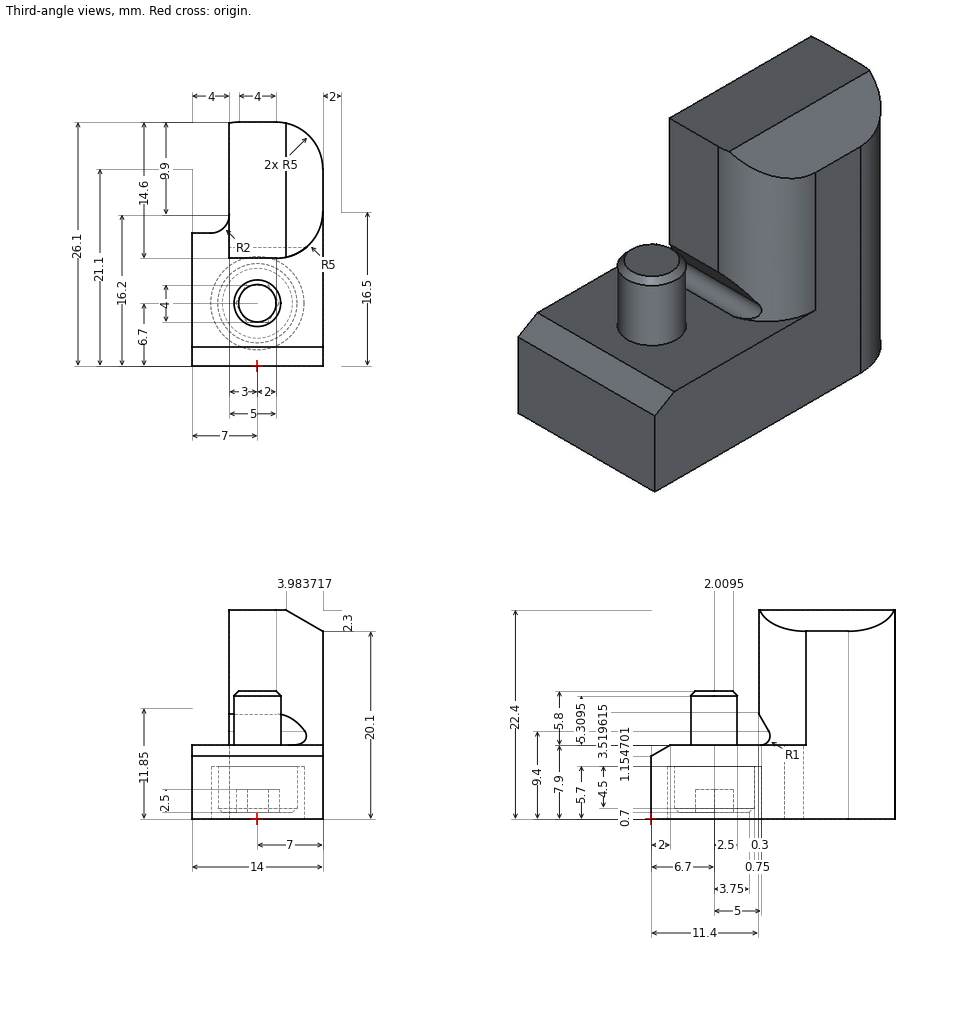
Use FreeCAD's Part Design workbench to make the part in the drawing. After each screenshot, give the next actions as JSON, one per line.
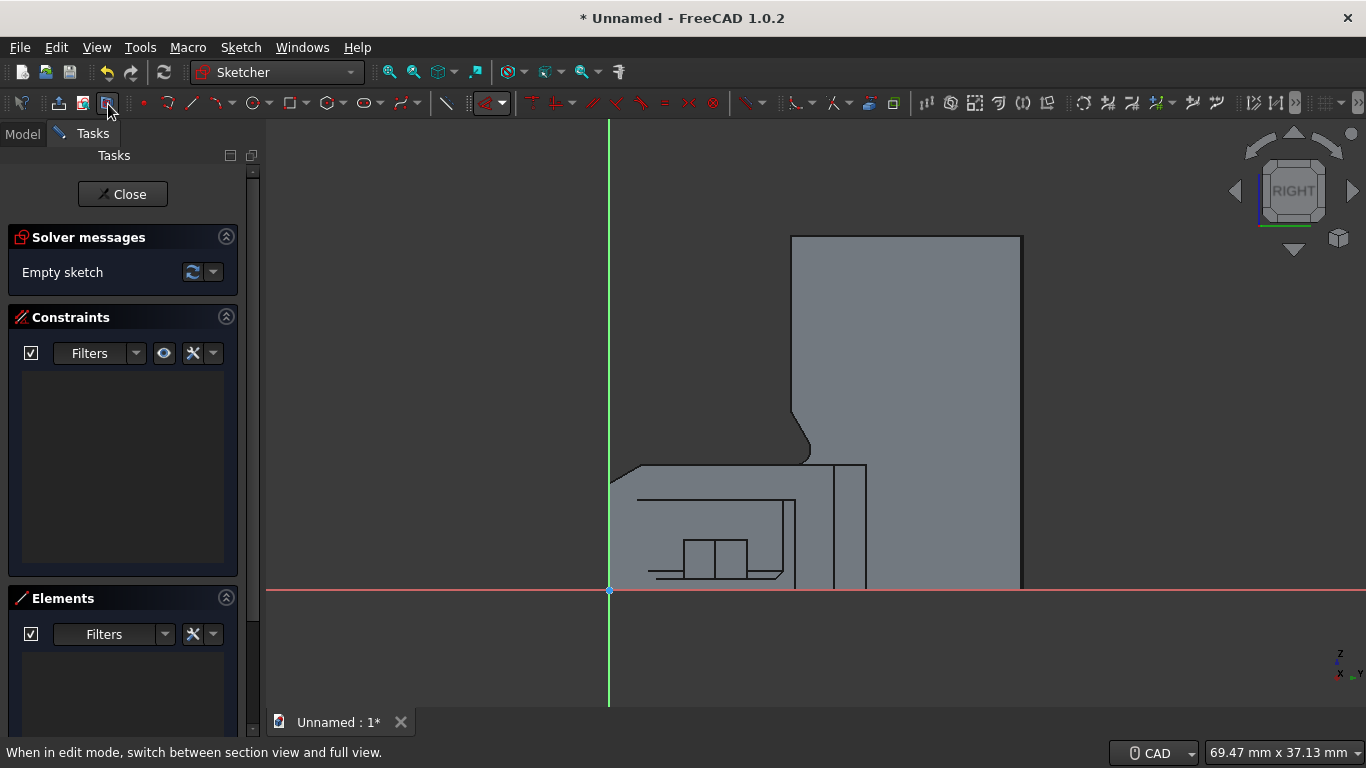
{"action": "scroll", "coordinate": [549, 566], "scroll_direction": "up", "scroll_amount": 2}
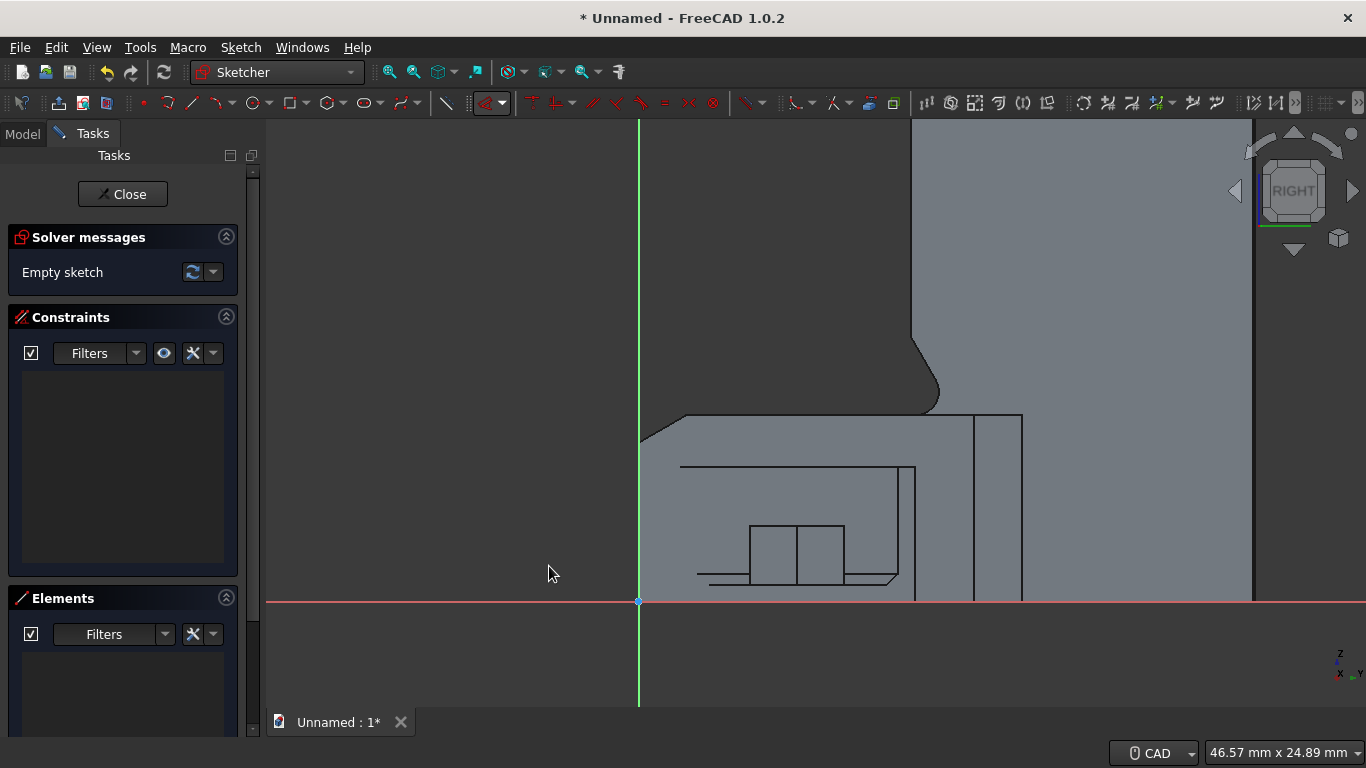
{"action": "left_click", "coordinate": [168, 104]}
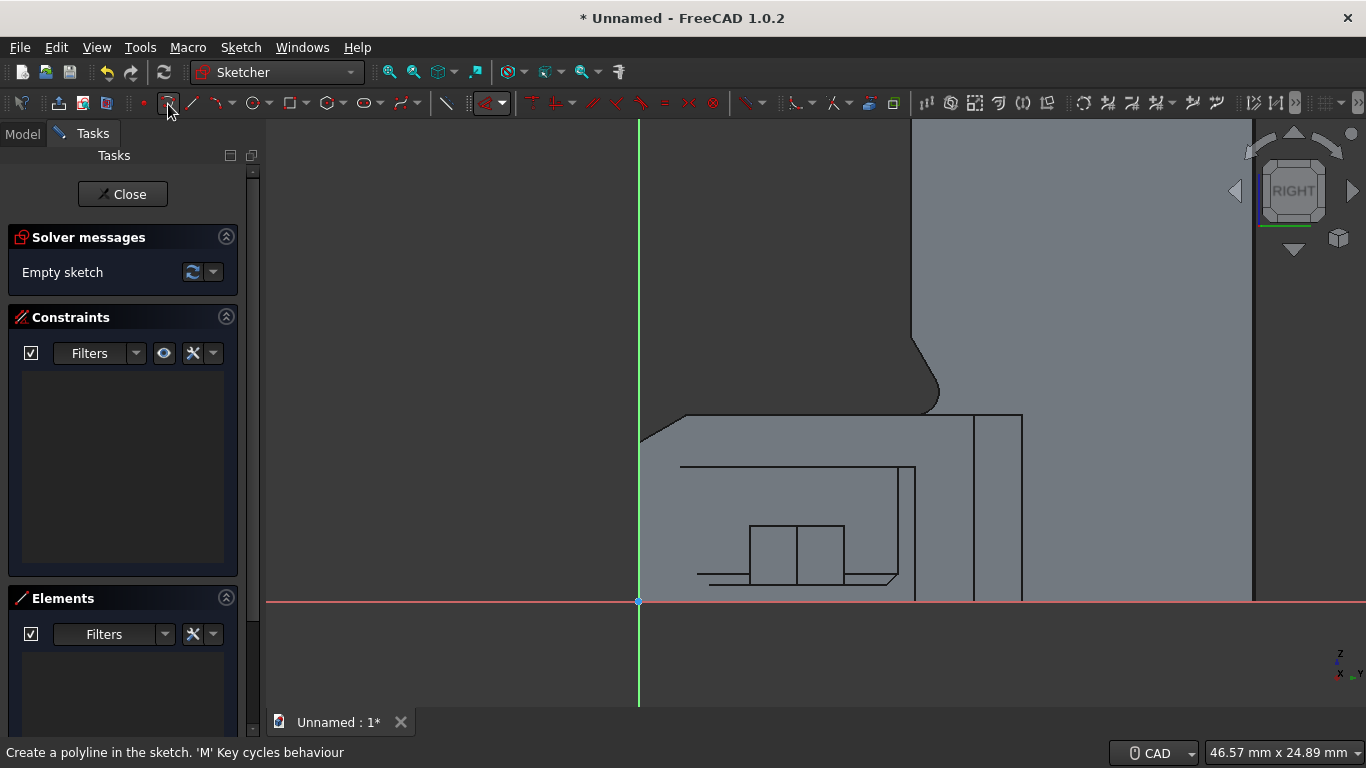
{"action": "left_click", "coordinate": [797, 415]}
{"action": "left_click", "coordinate": [856, 415]}
{"action": "left_click", "coordinate": [856, 290]}
{"action": "left_click", "coordinate": [845, 278]}
{"action": "left_click", "coordinate": [797, 278]}
{"action": "left_click", "coordinate": [797, 416]}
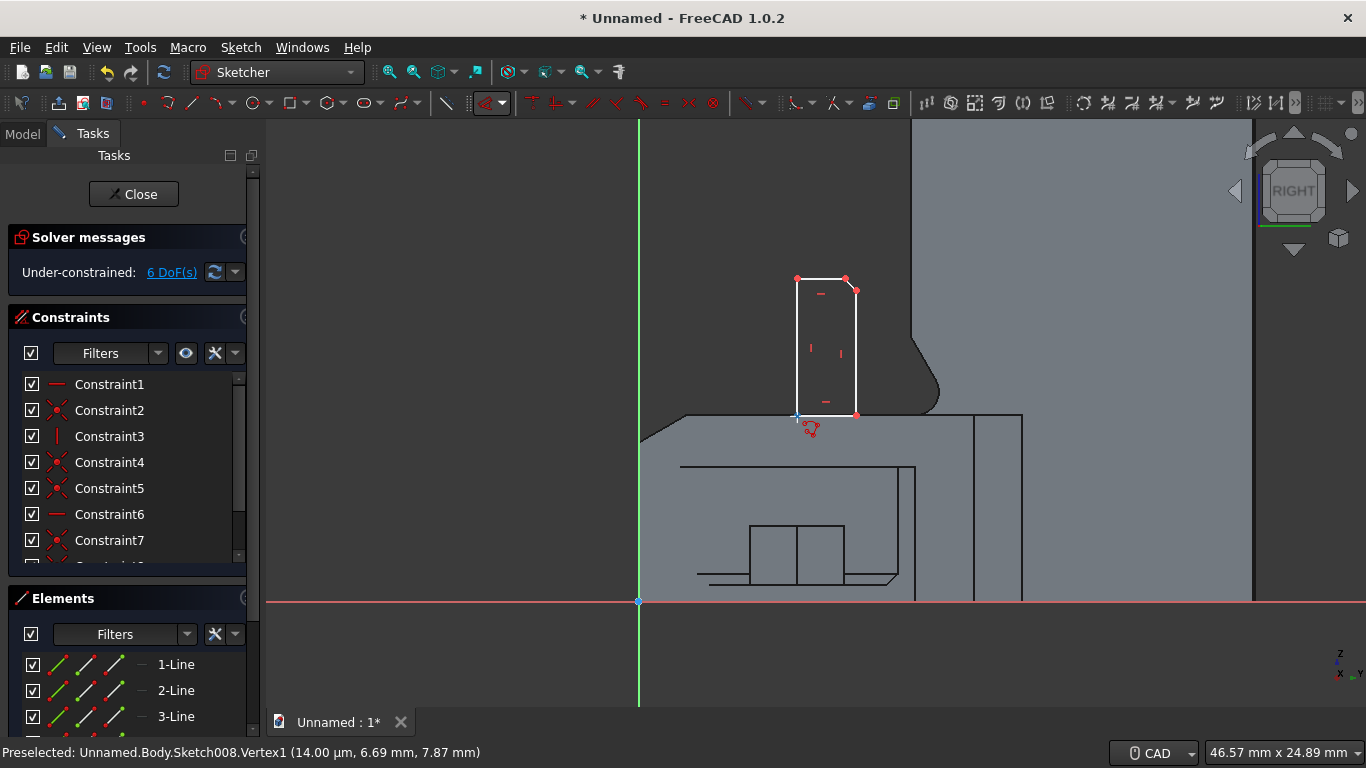
{"action": "left_click", "coordinate": [192, 104]}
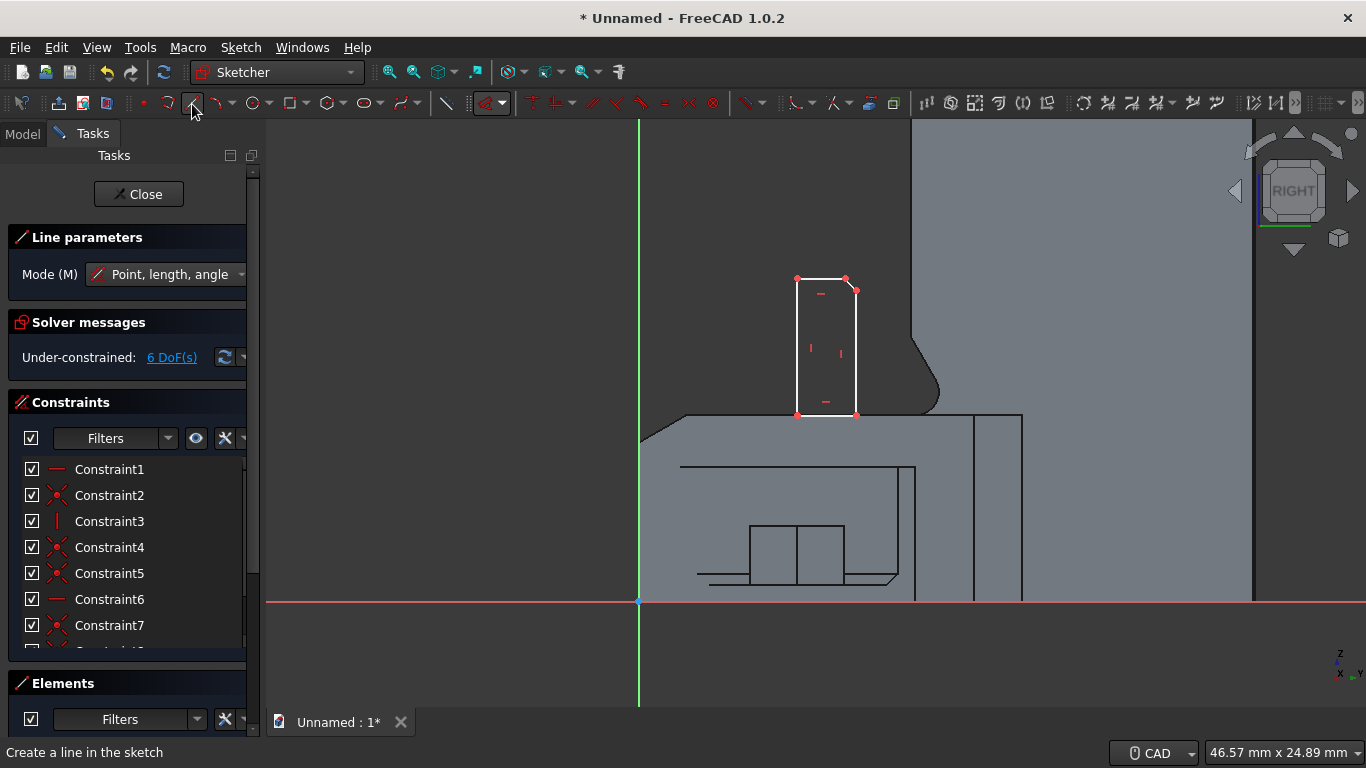
{"action": "left_click", "coordinate": [797, 265]}
{"action": "left_click", "coordinate": [797, 224]}
{"action": "key", "text": "Escape"}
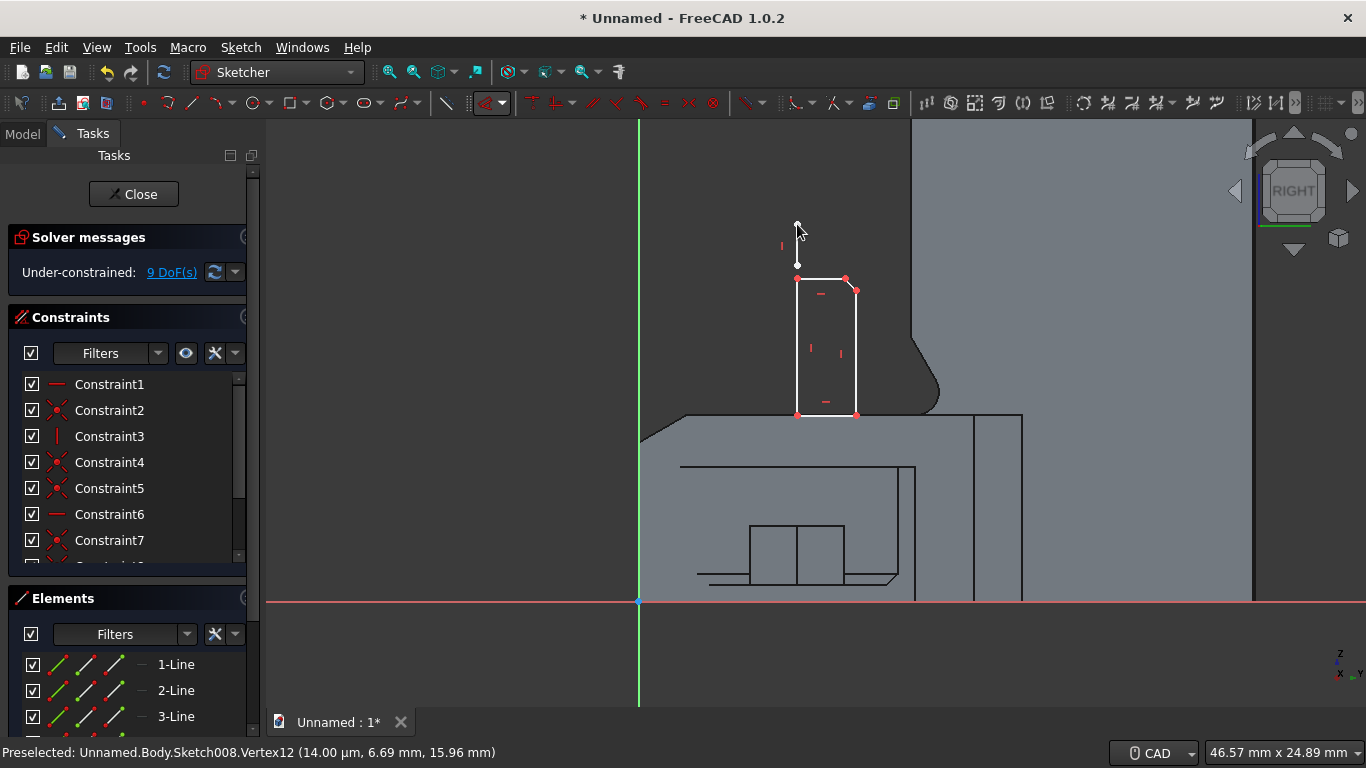
{"action": "left_click", "coordinate": [797, 254]}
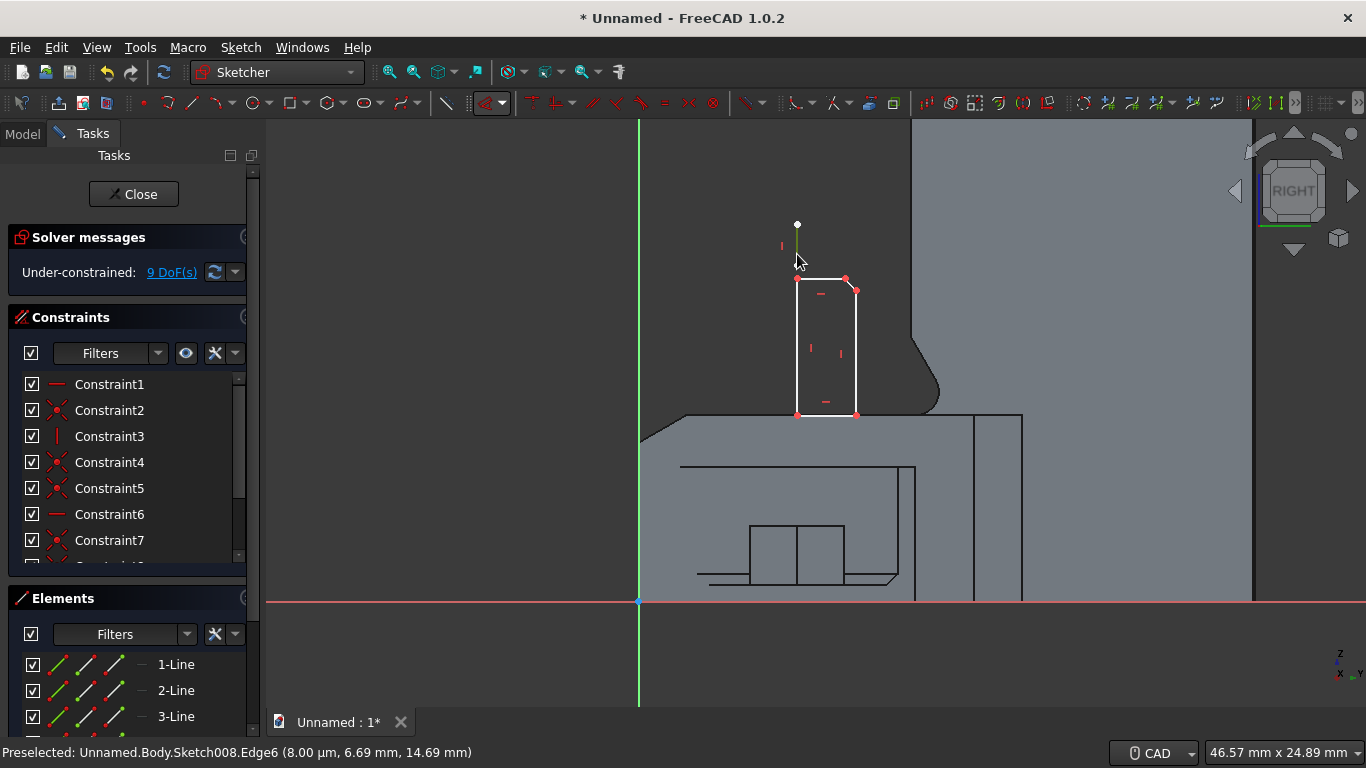
{"action": "left_click", "coordinate": [448, 104]}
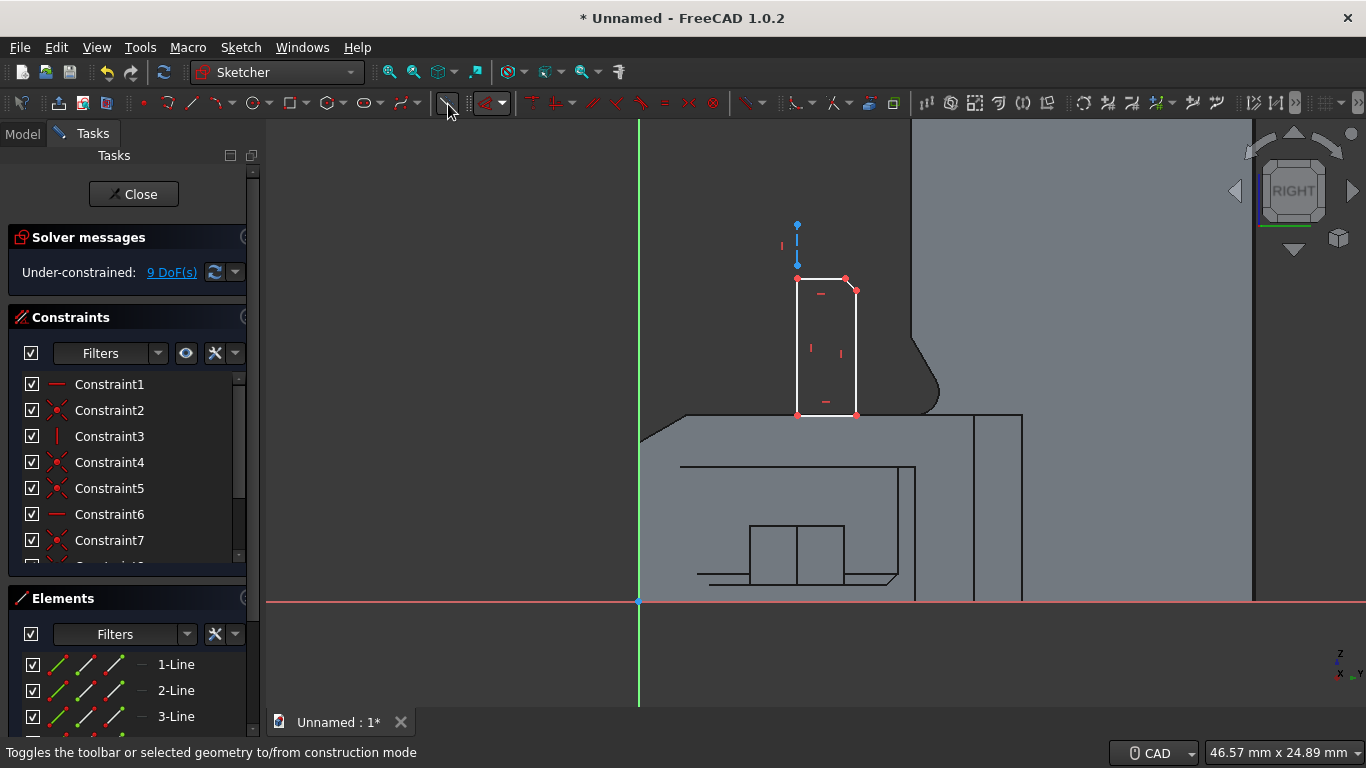
{"action": "left_click", "coordinate": [815, 416]}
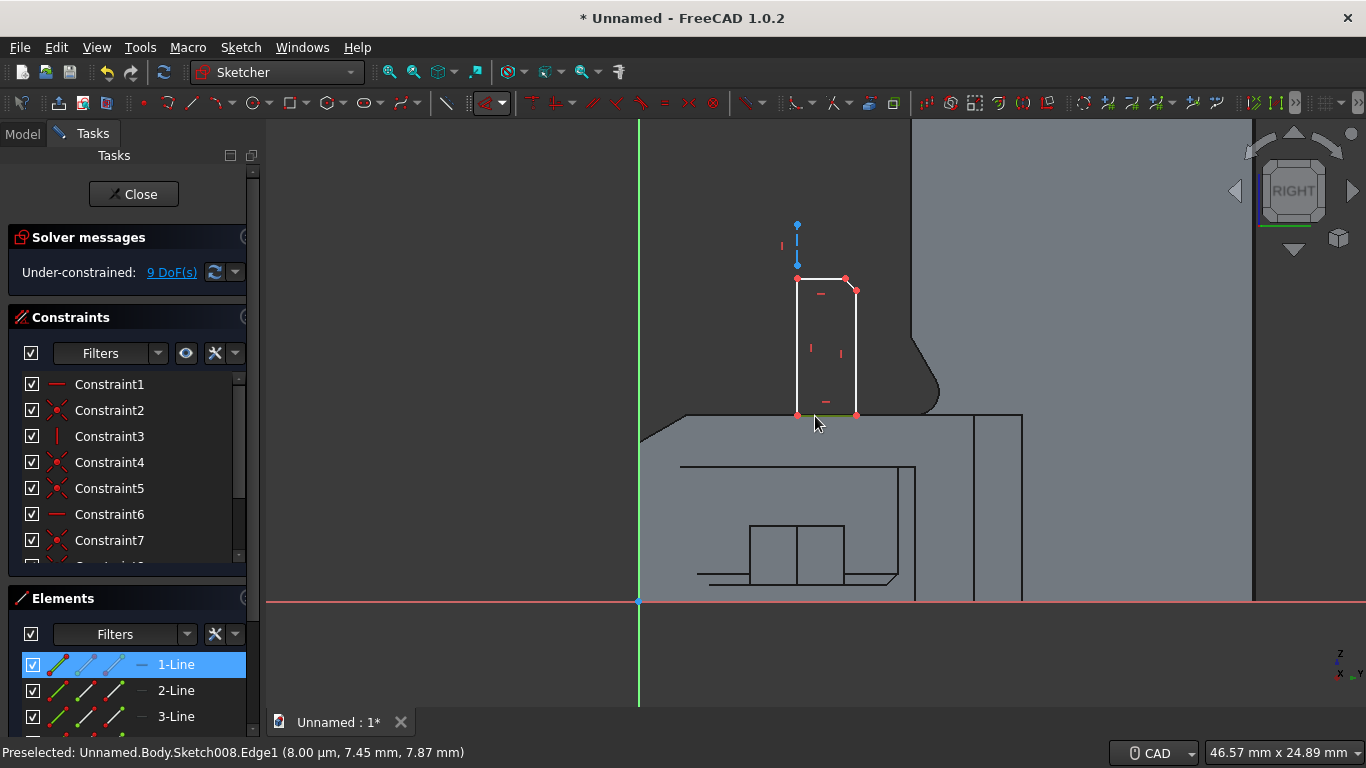
{"action": "key", "text": "l"}